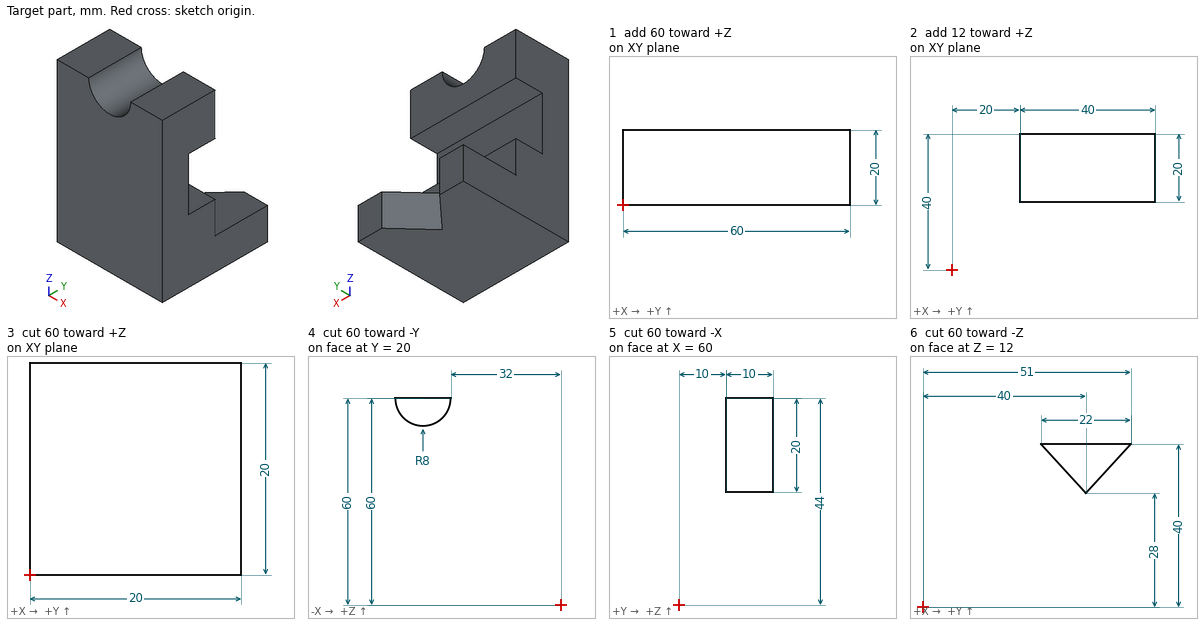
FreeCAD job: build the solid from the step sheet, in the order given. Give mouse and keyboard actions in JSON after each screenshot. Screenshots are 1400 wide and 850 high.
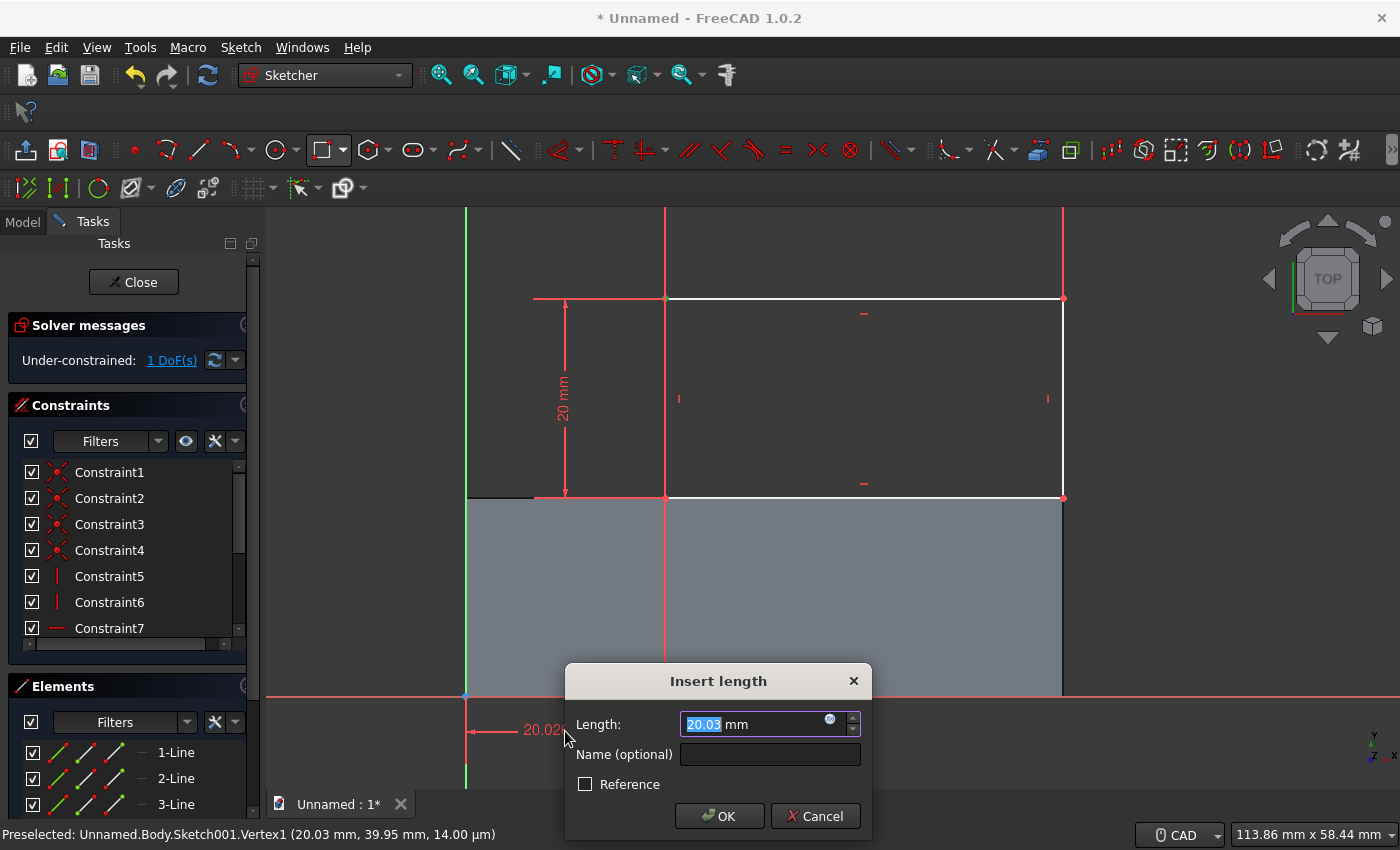
{"action": "type", "text": "20"}
{"action": "key", "text": "Return"}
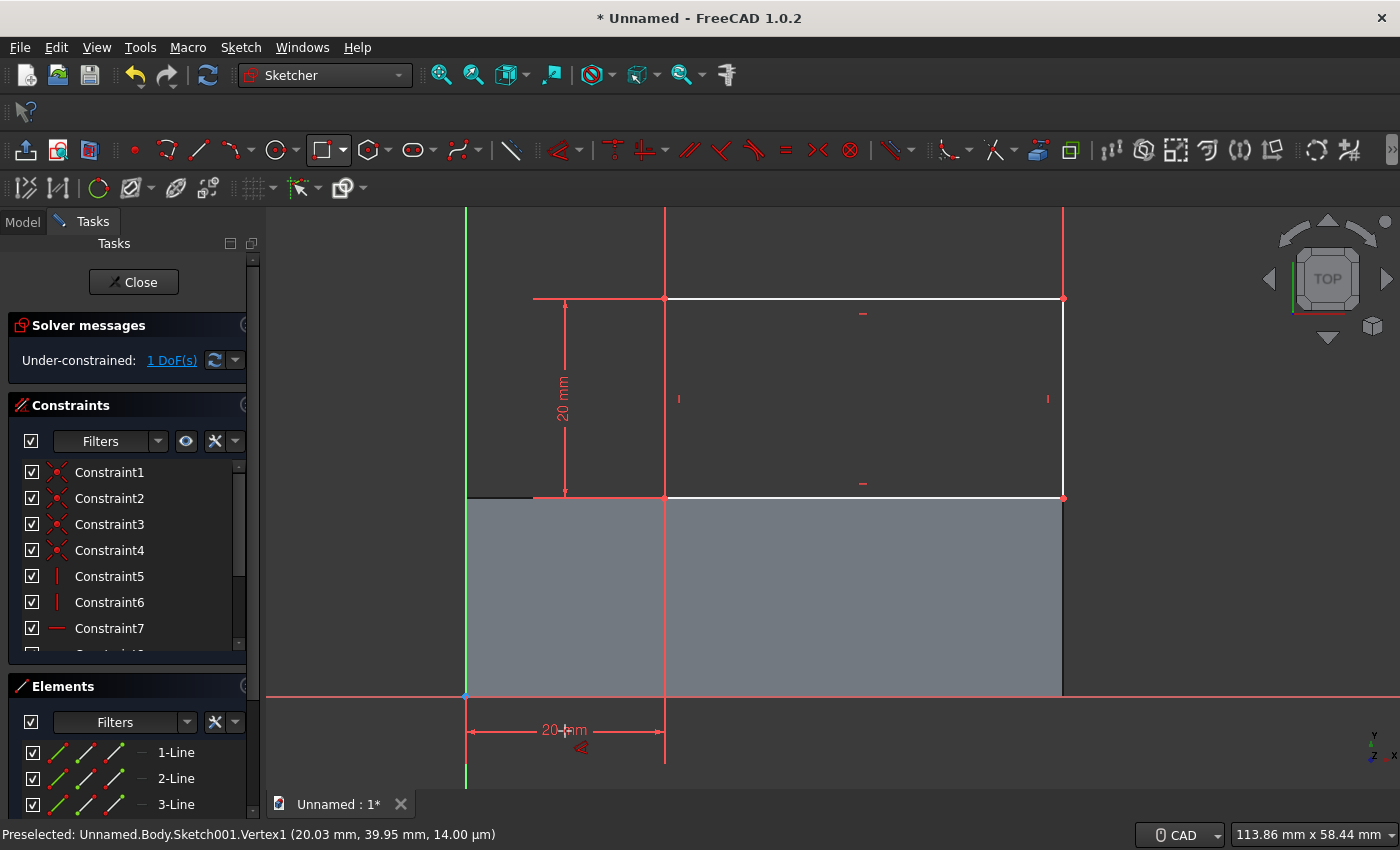
{"action": "left_click", "coordinate": [665, 299]}
{"action": "left_click", "coordinate": [432, 498]}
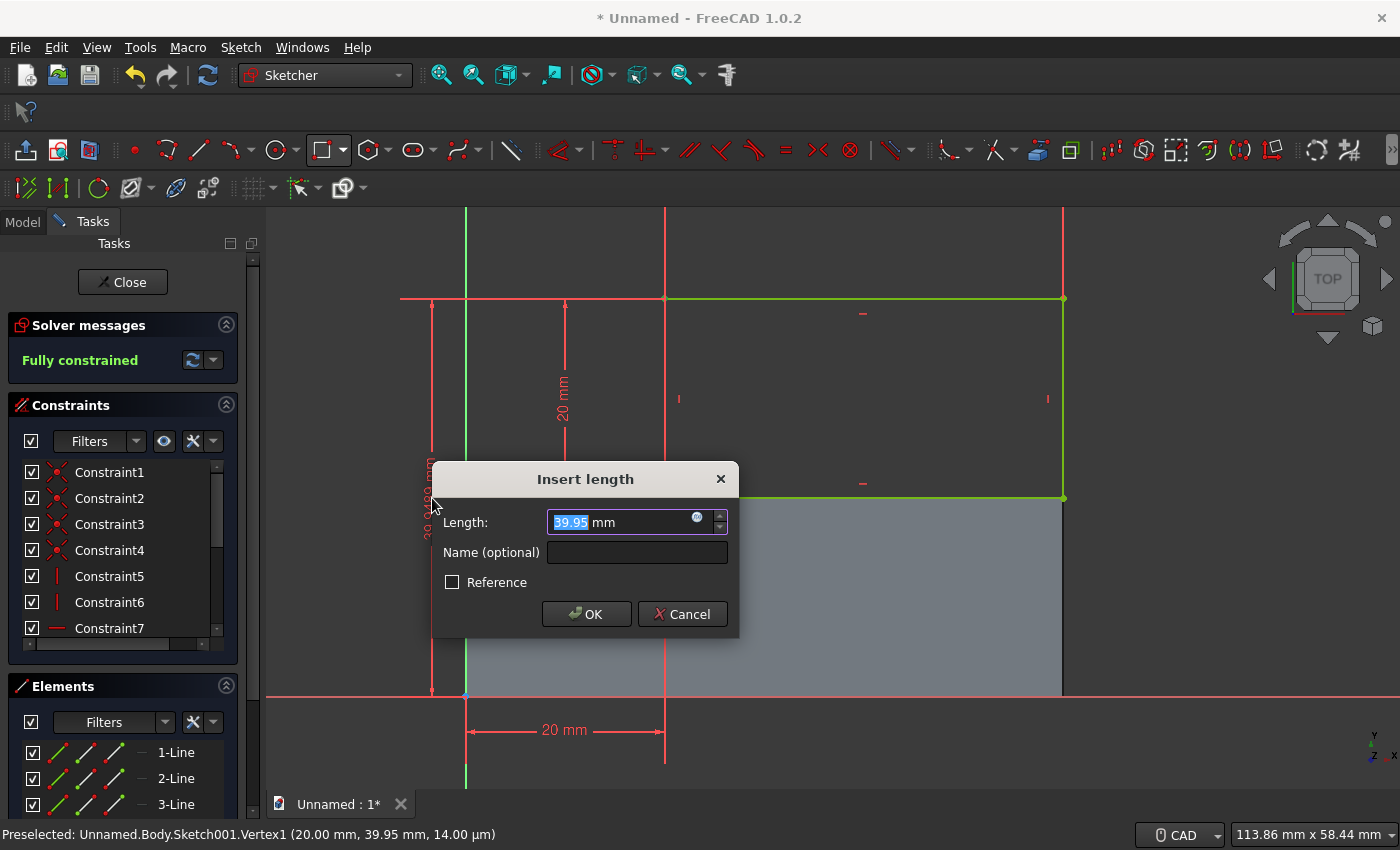
{"action": "type", "text": "40"}
{"action": "key", "text": "Return"}
{"action": "key", "text": "Escape"}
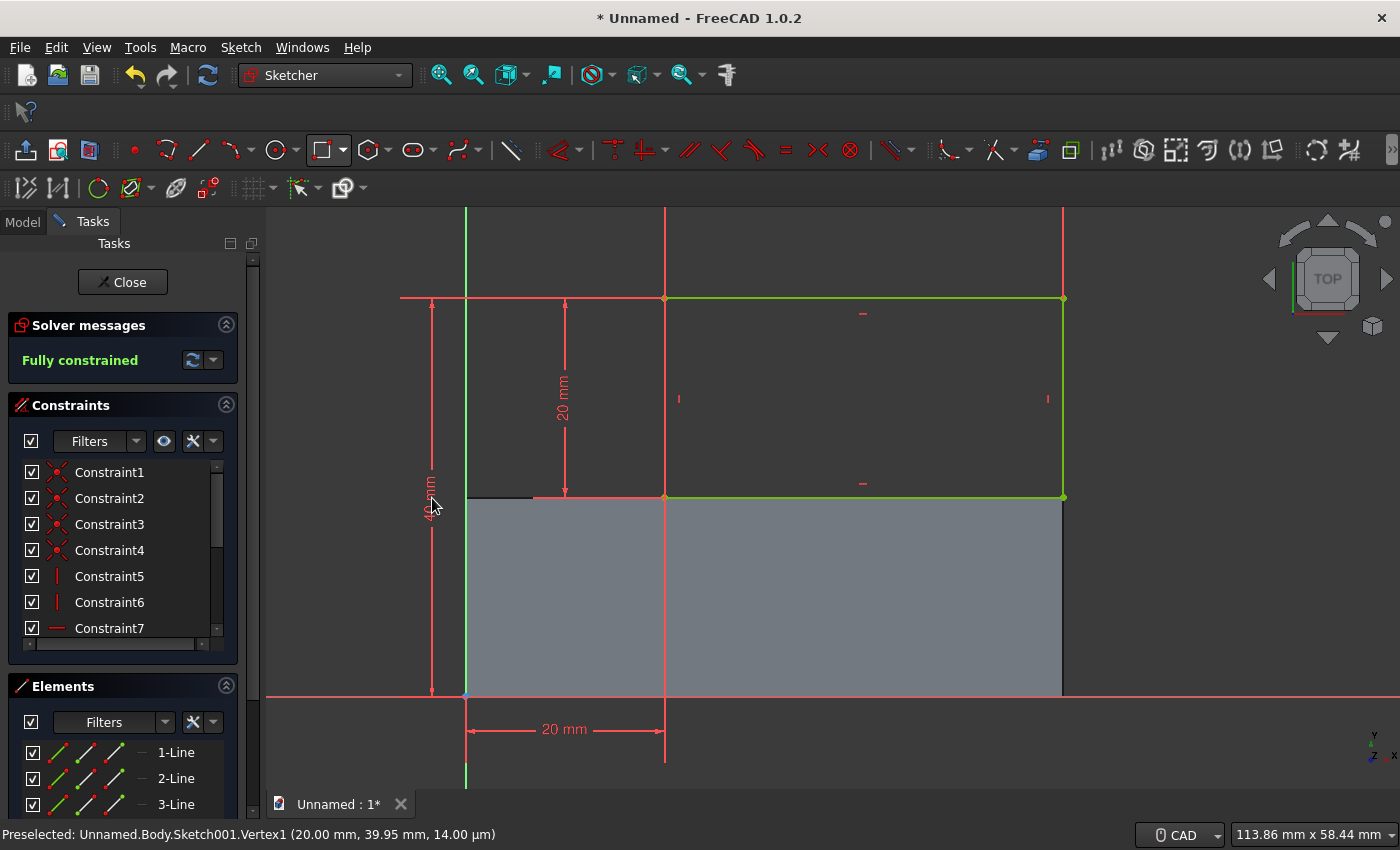
{"action": "left_click", "coordinate": [123, 282]}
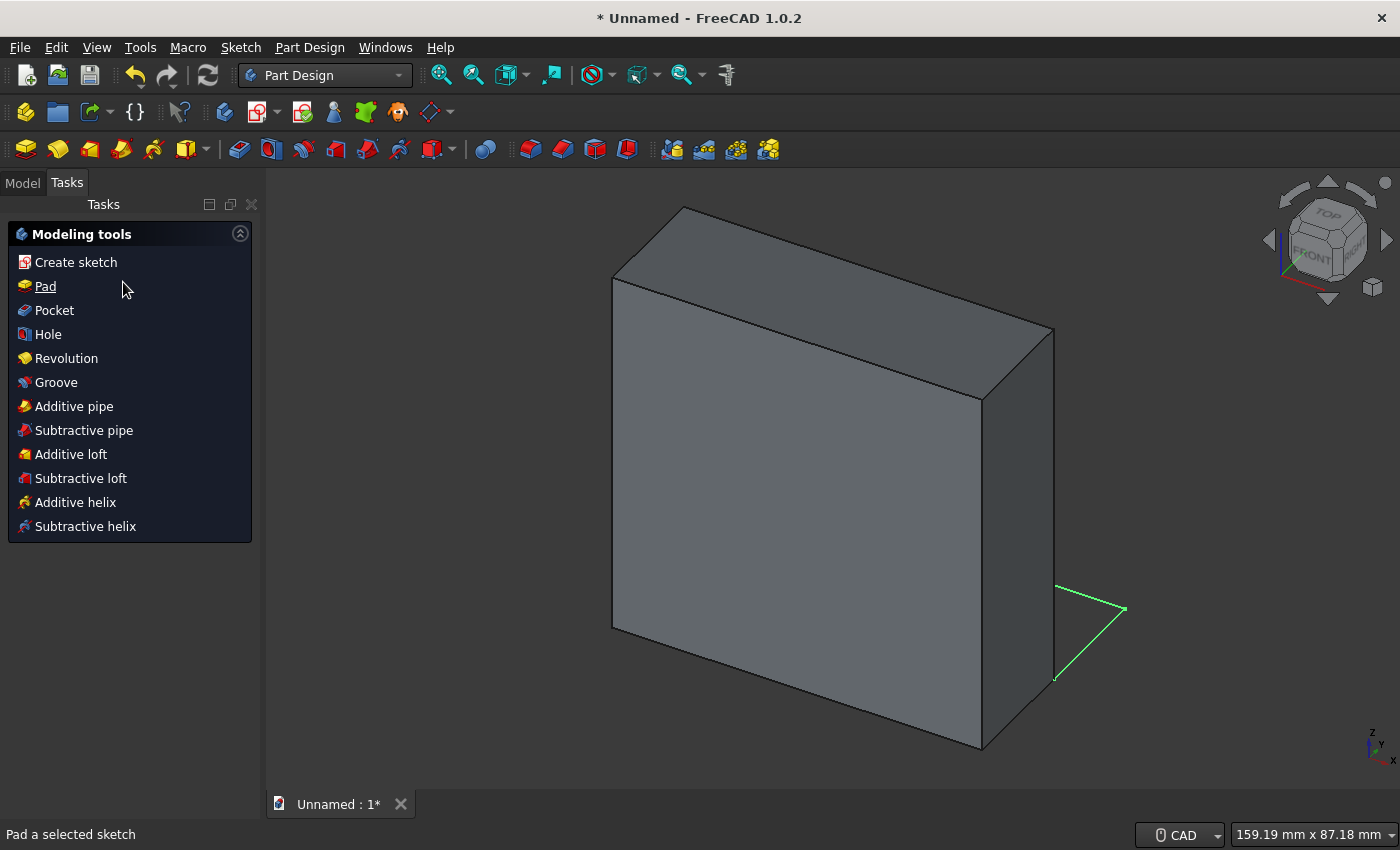
{"action": "left_click", "coordinate": [26, 150]}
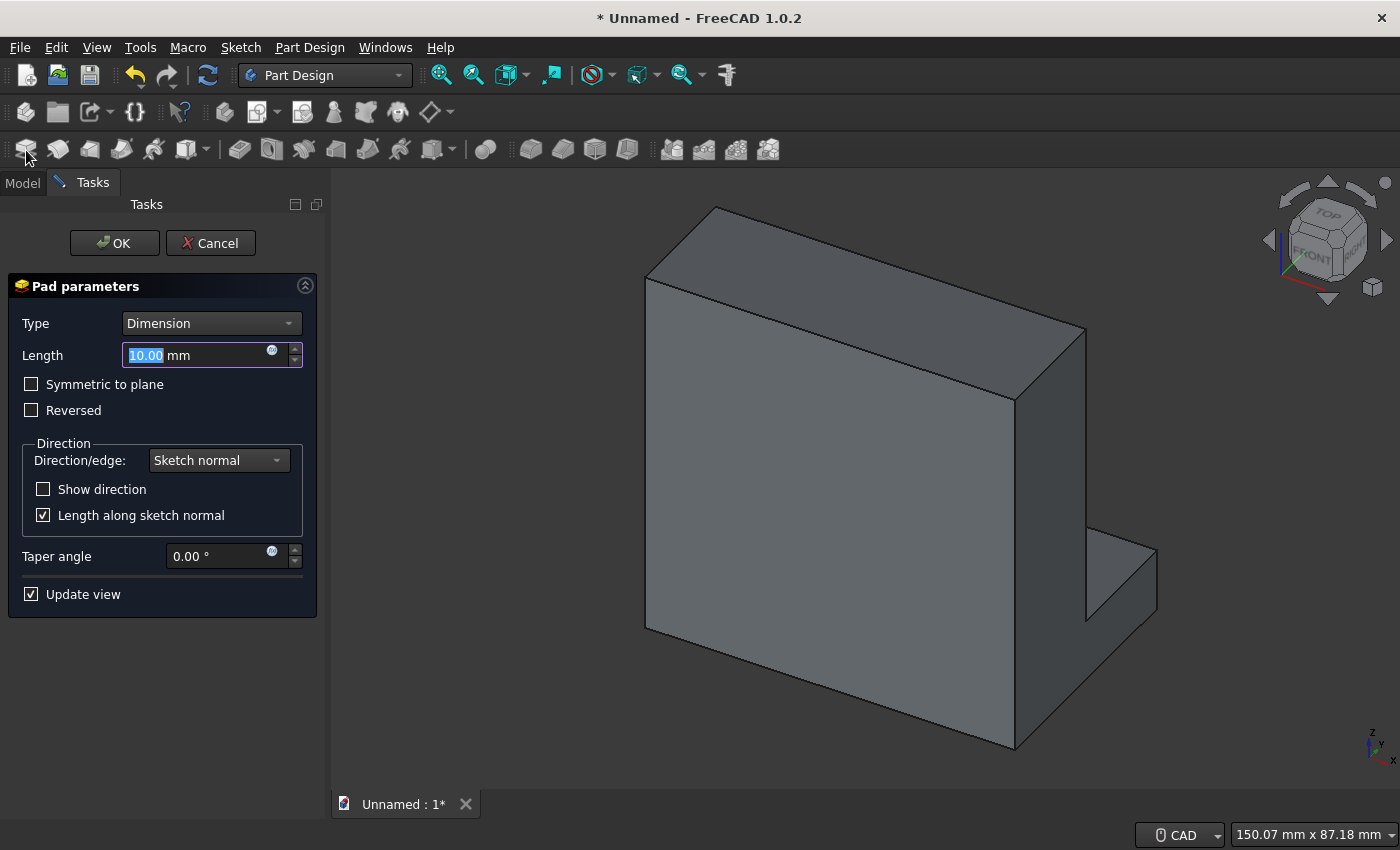
{"action": "type", "text": "12"}
{"action": "key", "text": "Tab"}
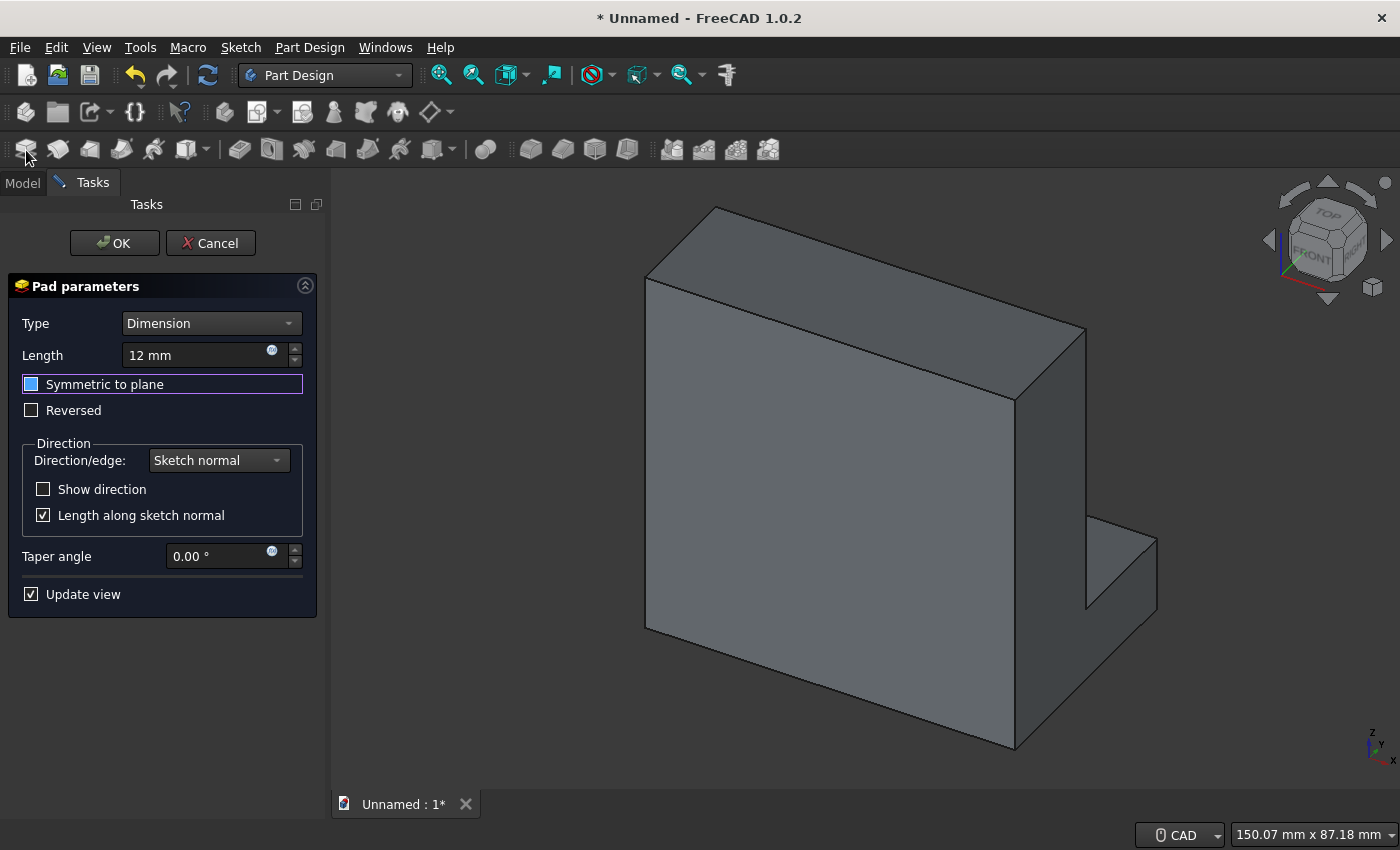
{"action": "left_click", "coordinate": [115, 243]}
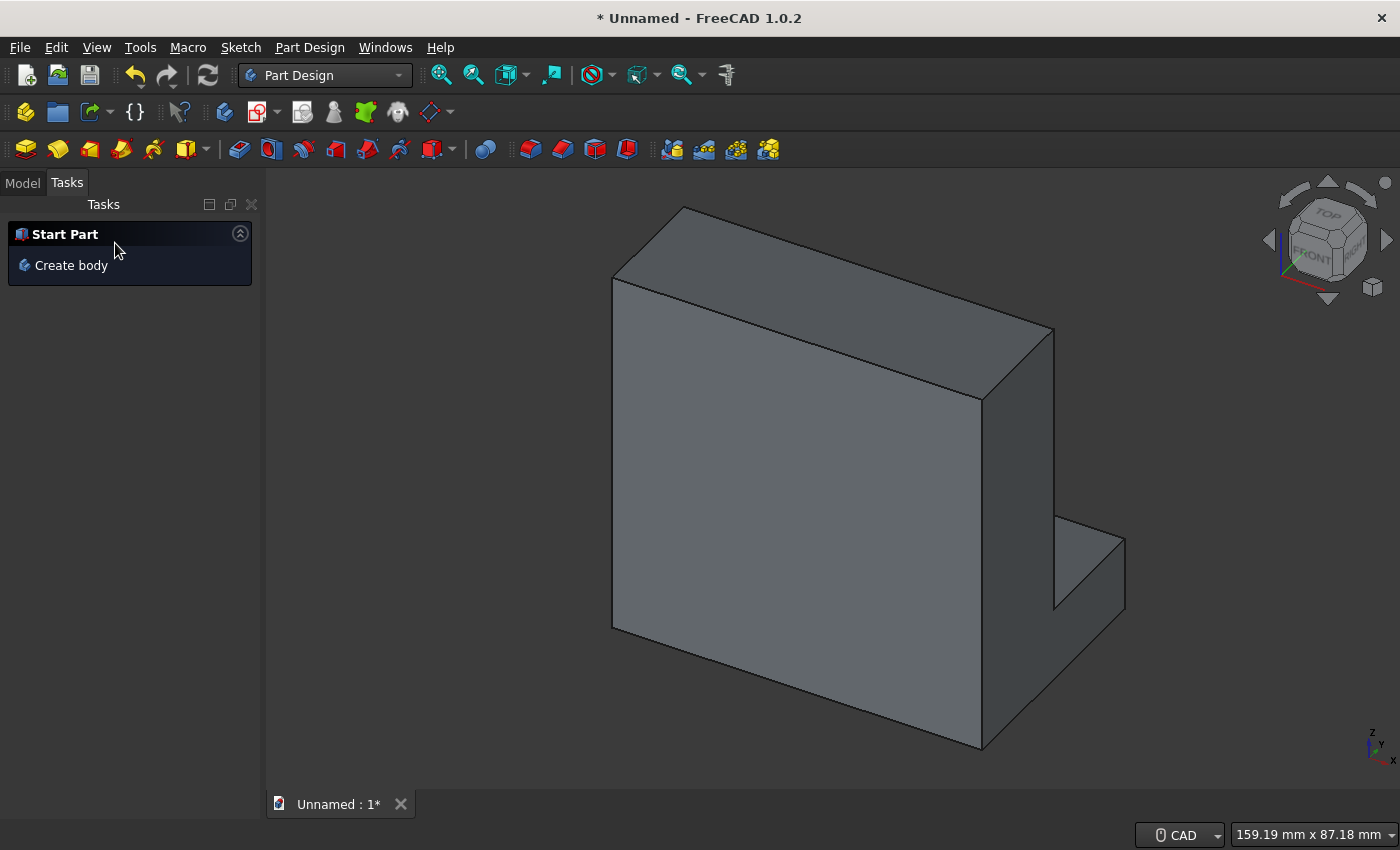
{"action": "key", "text": "v f"}